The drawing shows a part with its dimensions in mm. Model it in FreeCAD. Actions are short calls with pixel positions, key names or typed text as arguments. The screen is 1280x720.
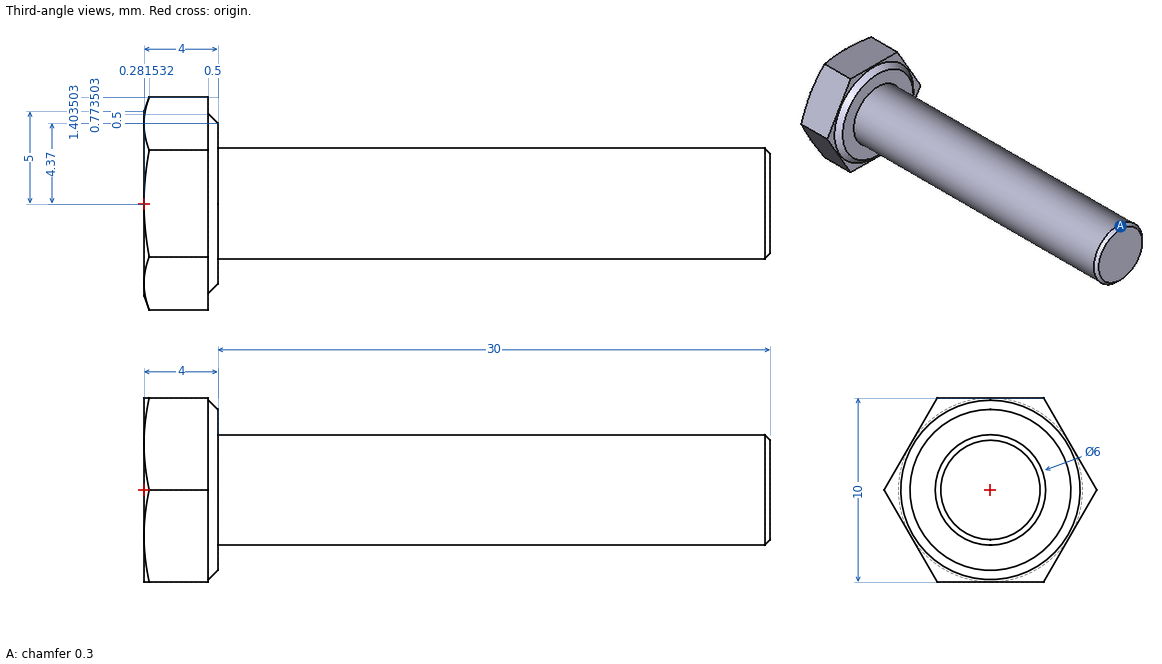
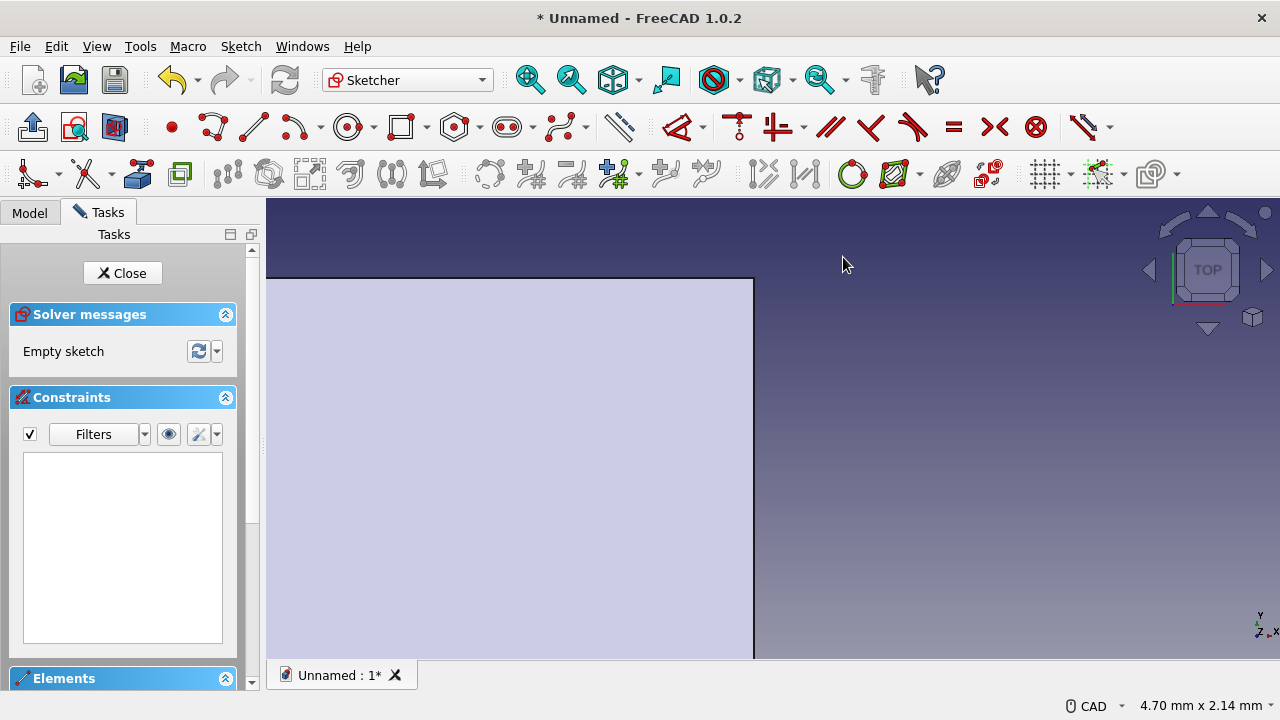
click(213, 128)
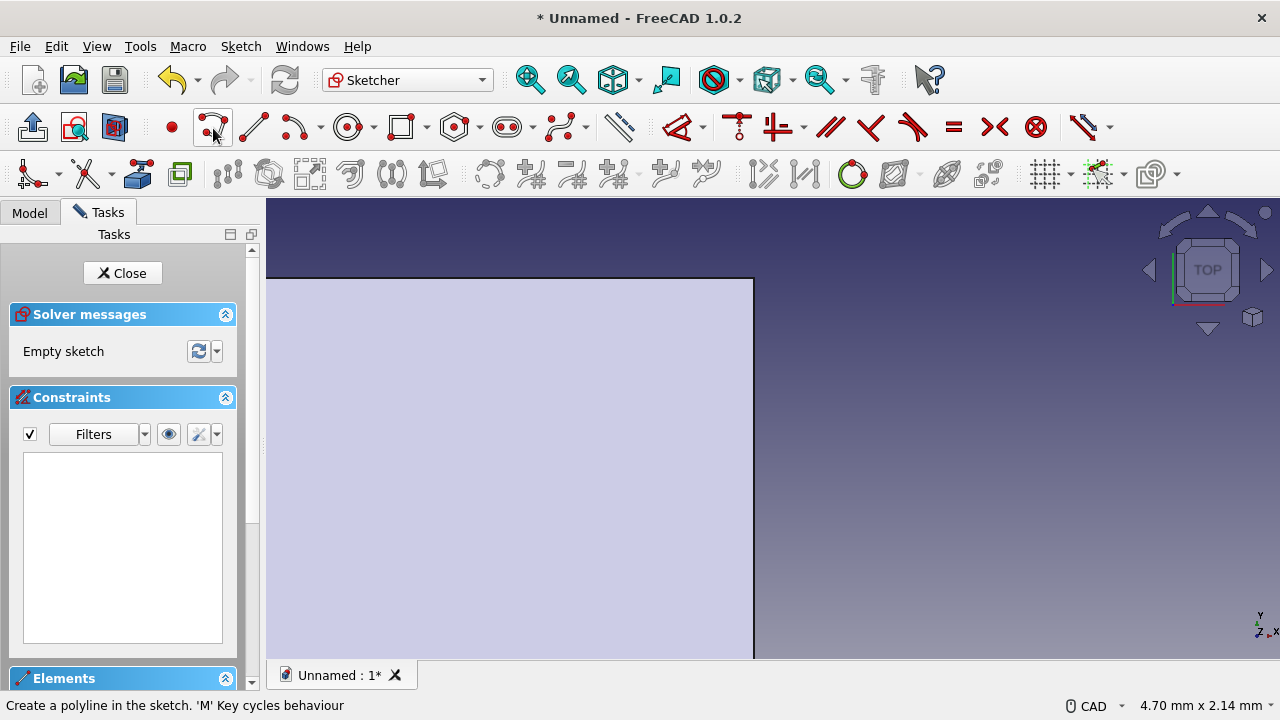
click(754, 581)
click(754, 278)
click(646, 278)
click(646, 473)
click(754, 582)
key(Escape)
key(Escape)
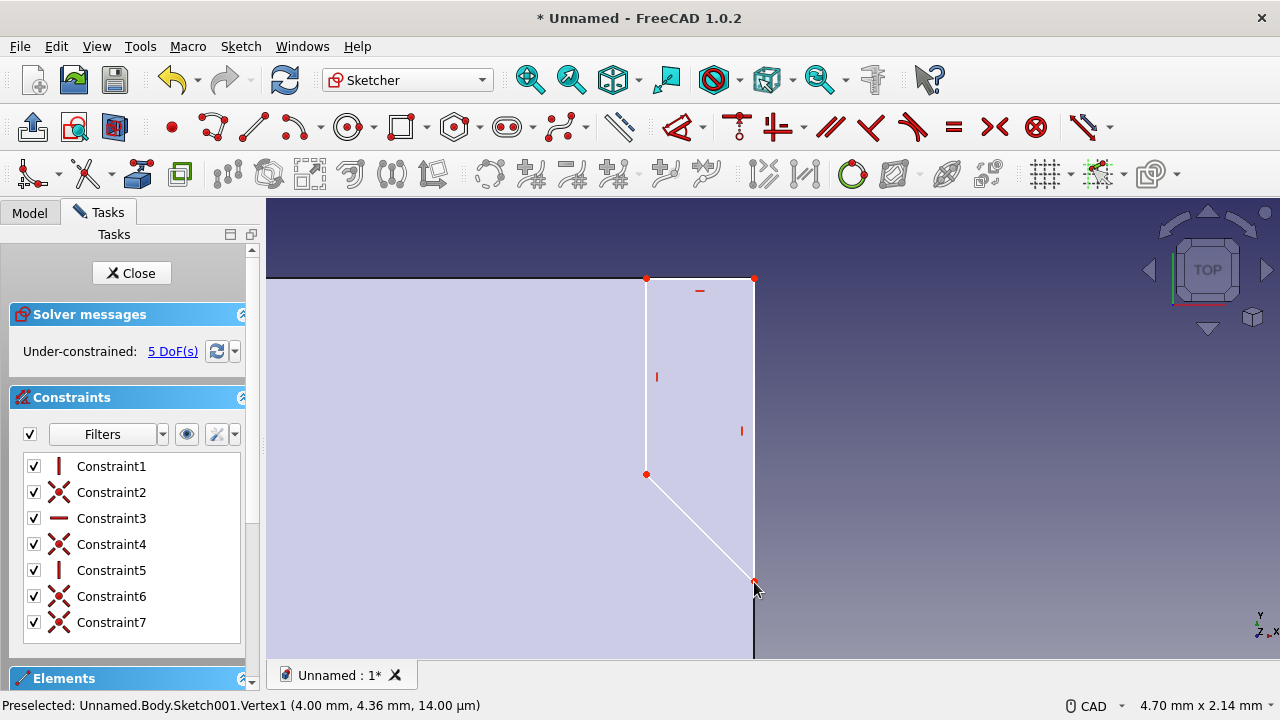
click(676, 128)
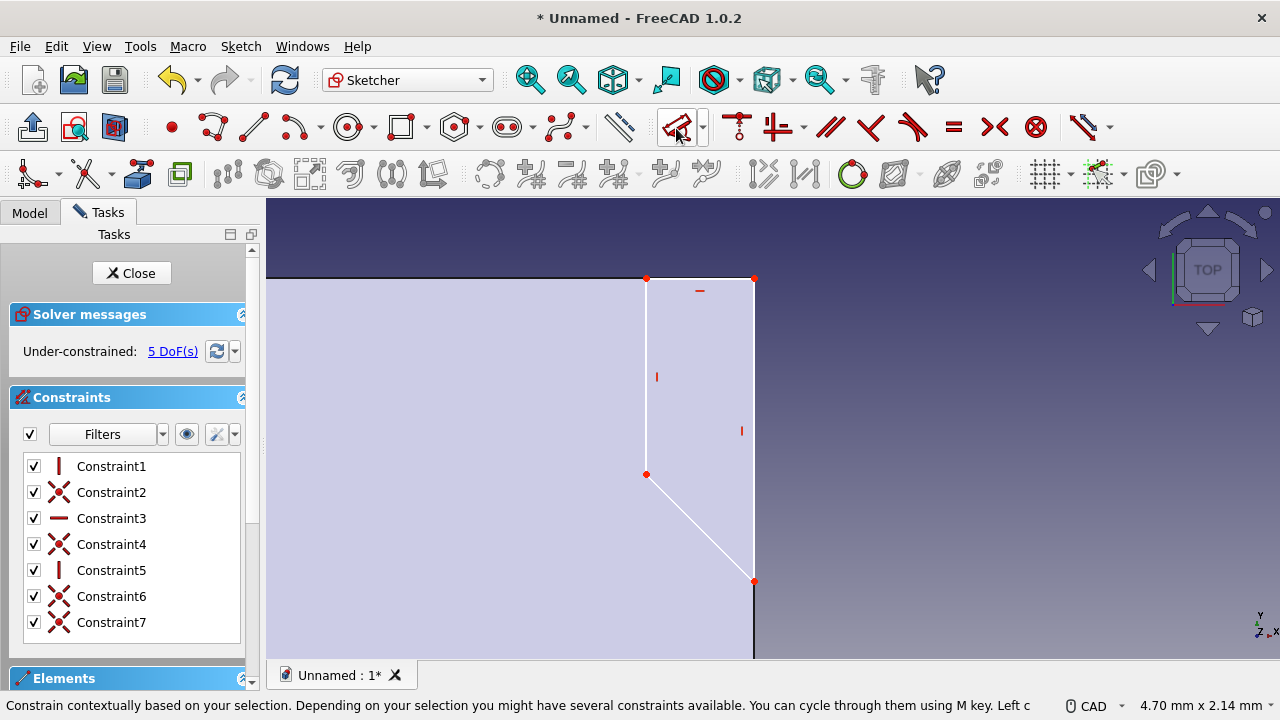
click(754, 582)
click(524, 548)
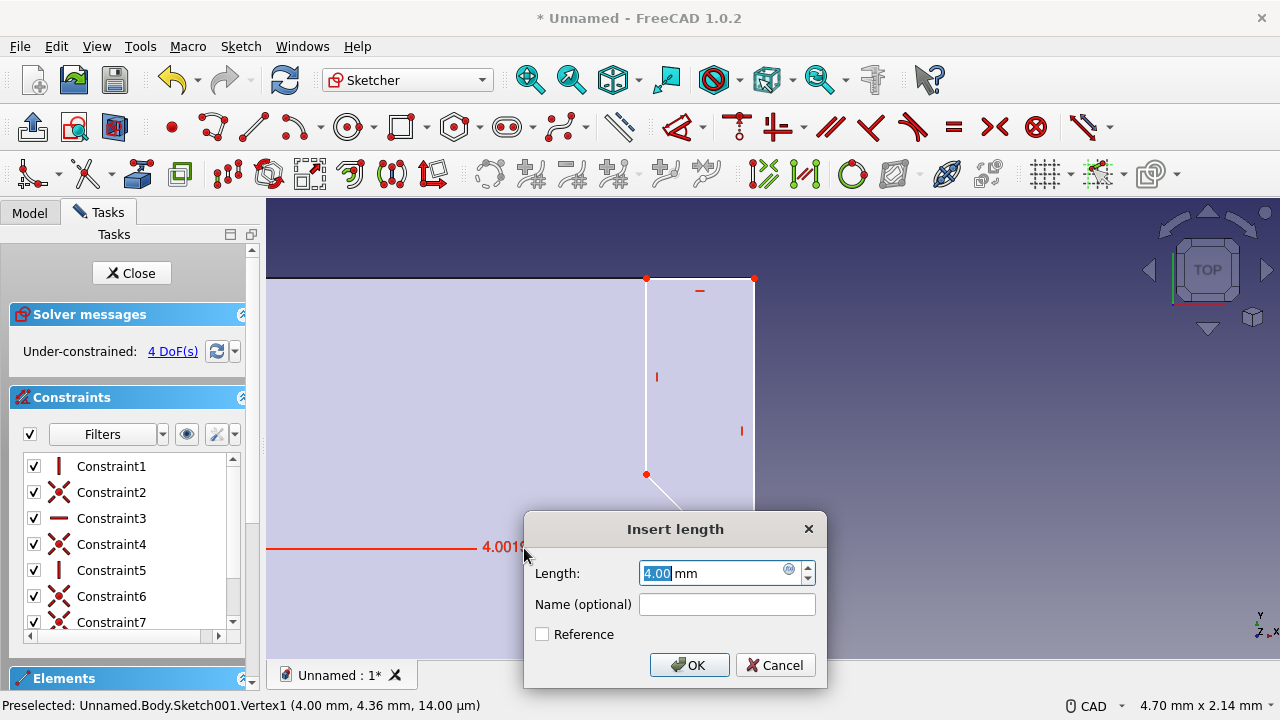
text(4)
key(Return)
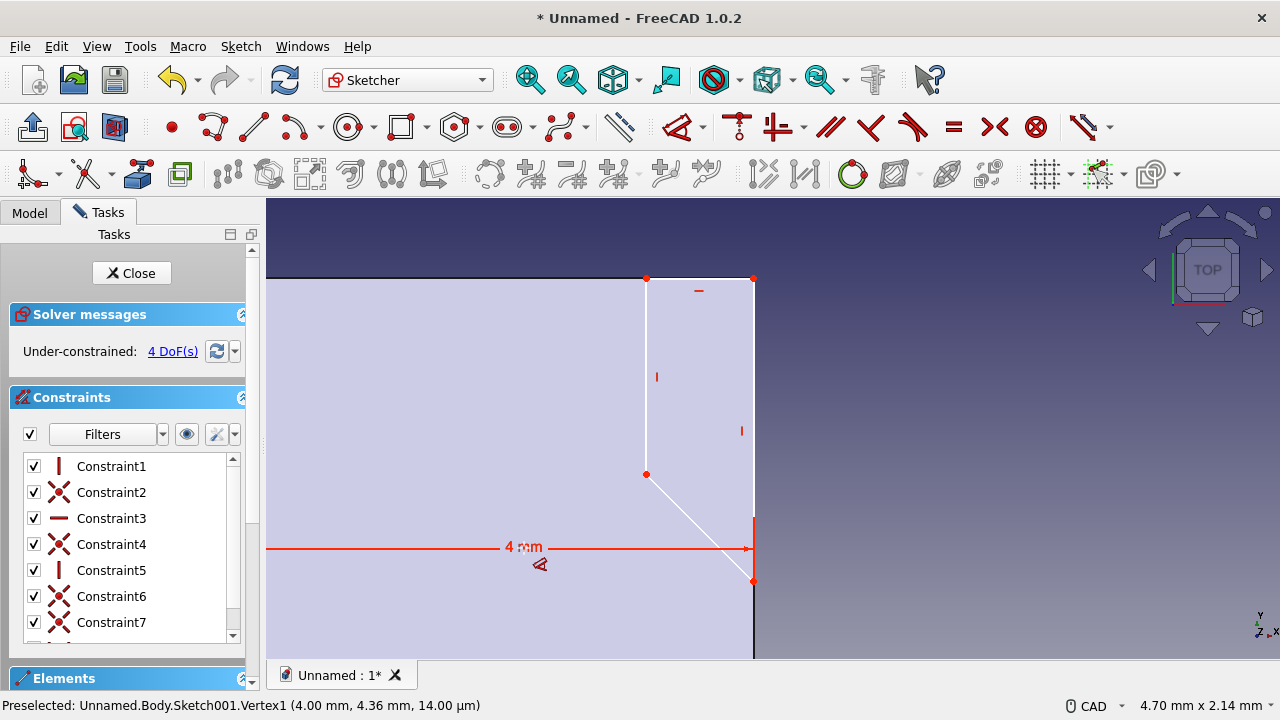
click(721, 279)
click(700, 245)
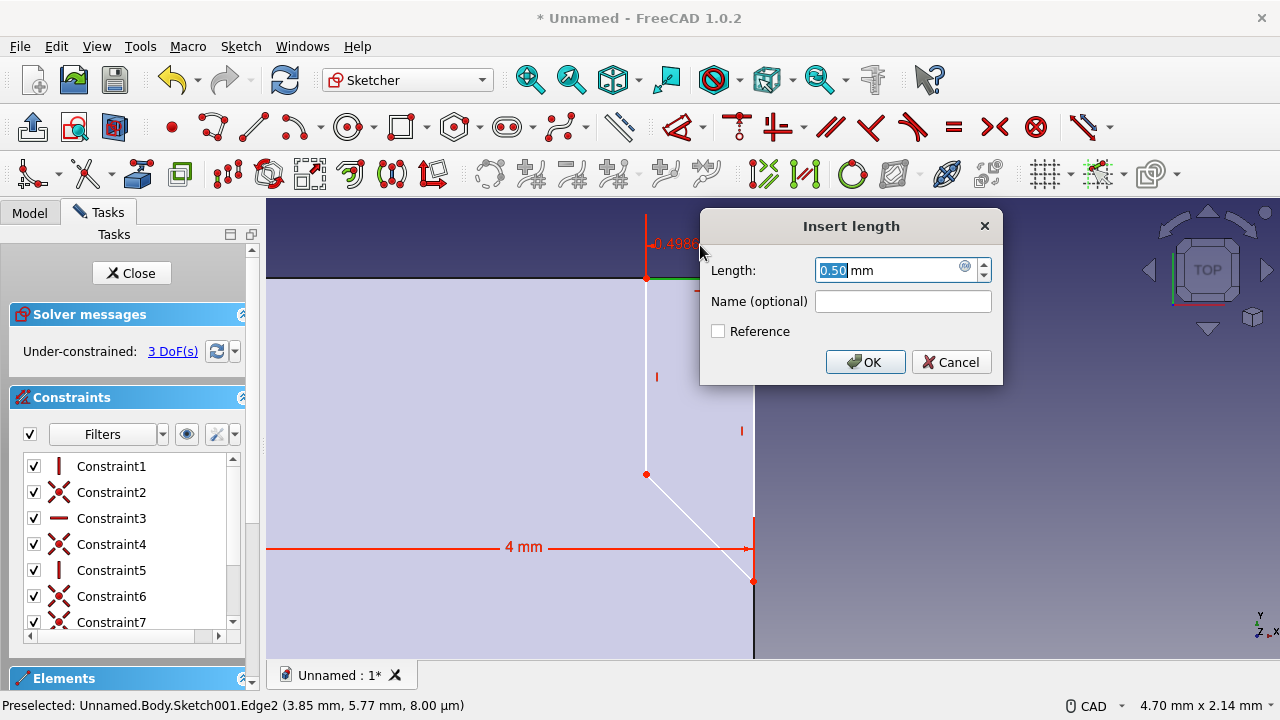
text(0.5)
key(Return)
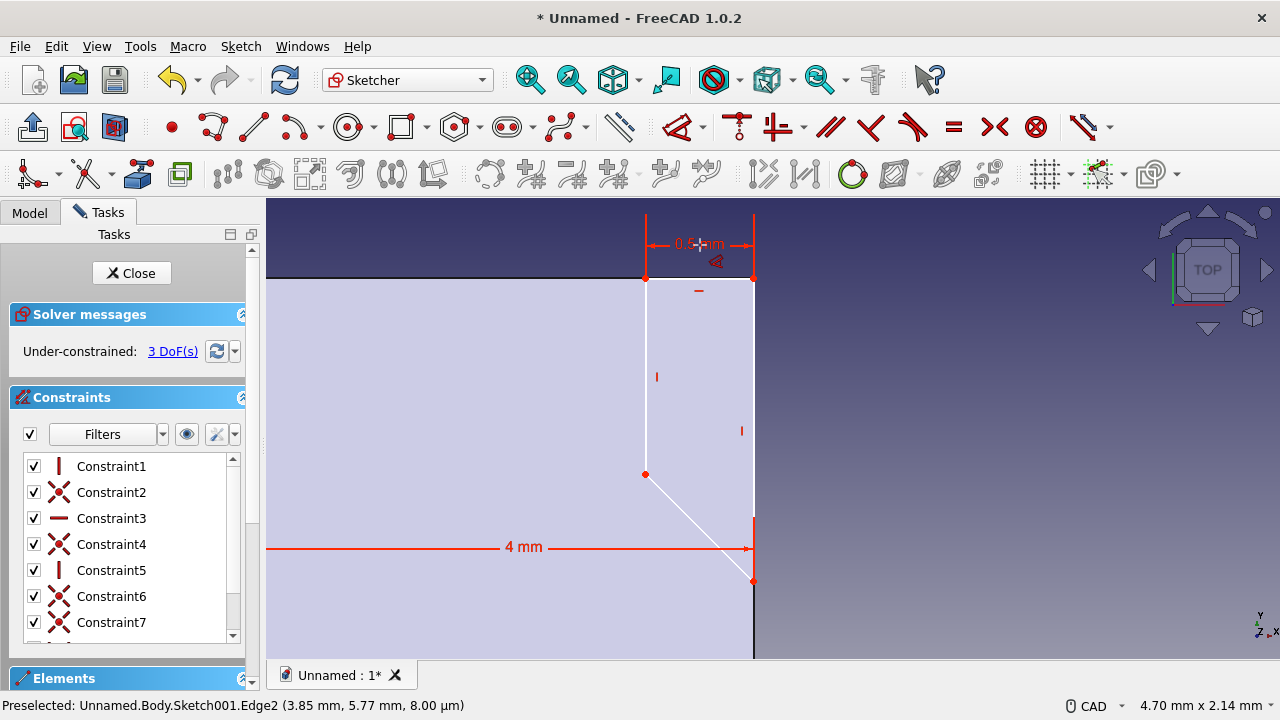
click(678, 506)
click(788, 528)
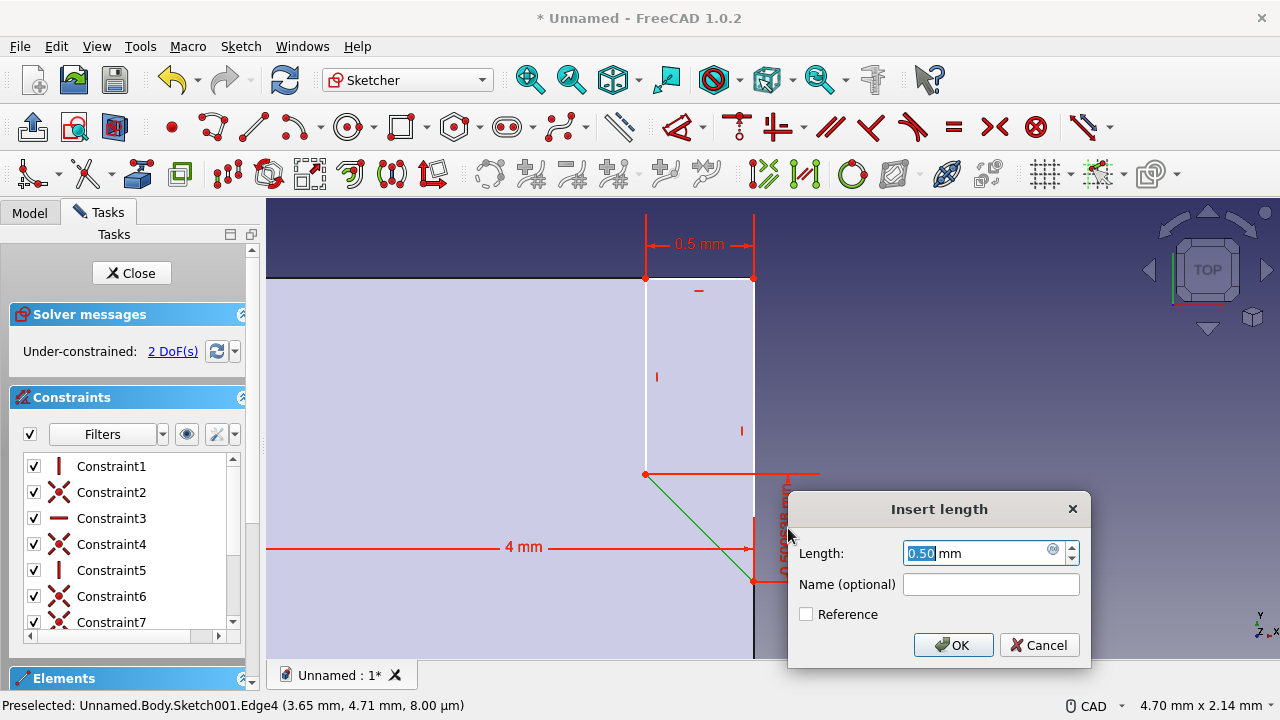
text(0.5)
key(Return)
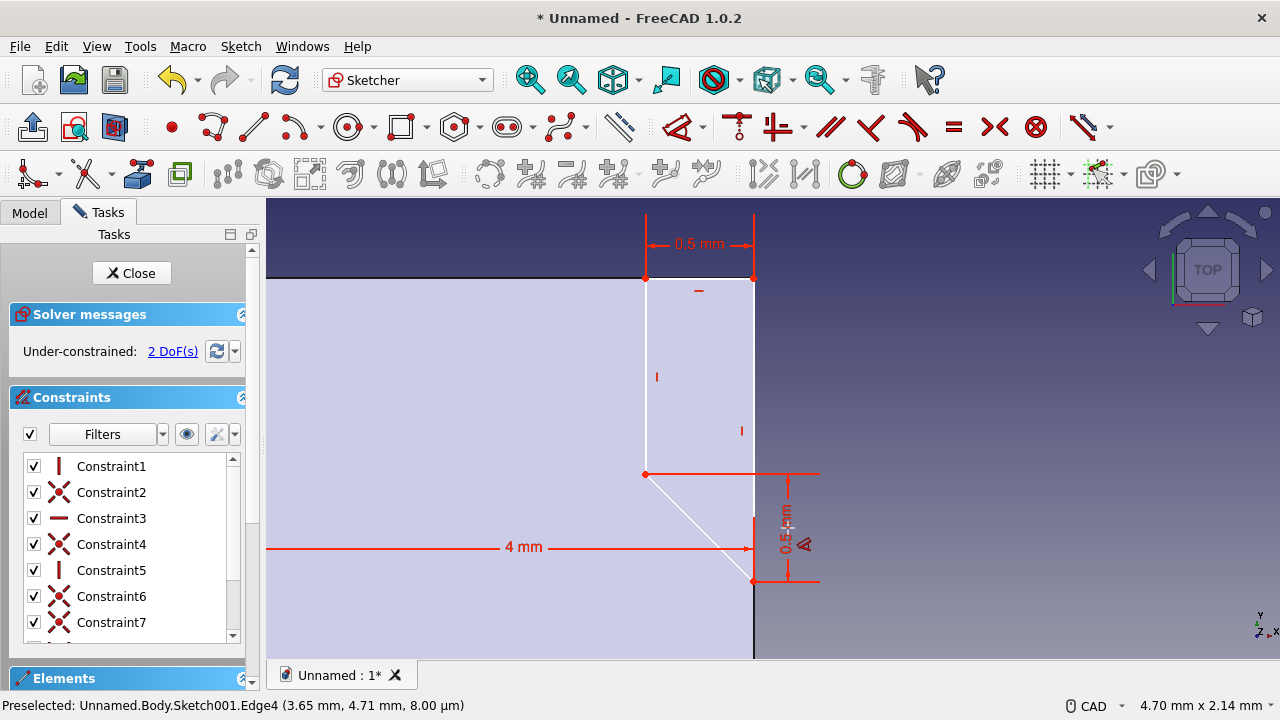
click(754, 582)
click(788, 607)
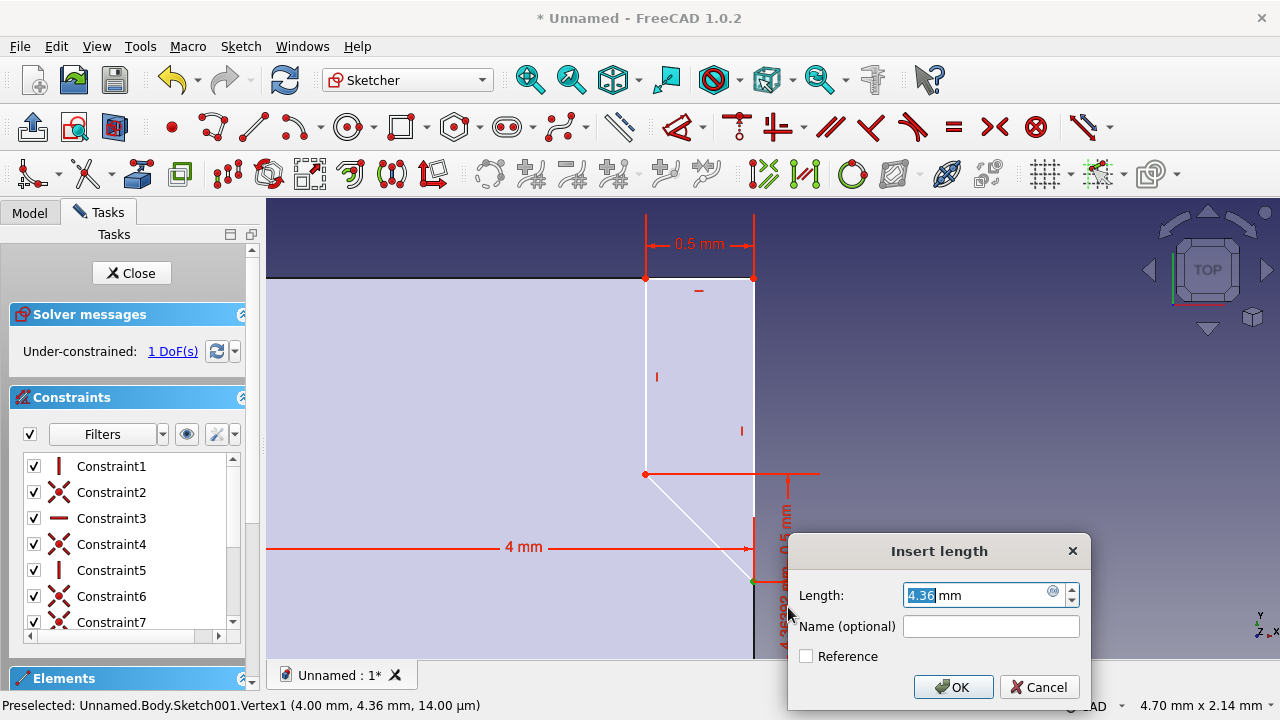
text(4.37)
key(Return)